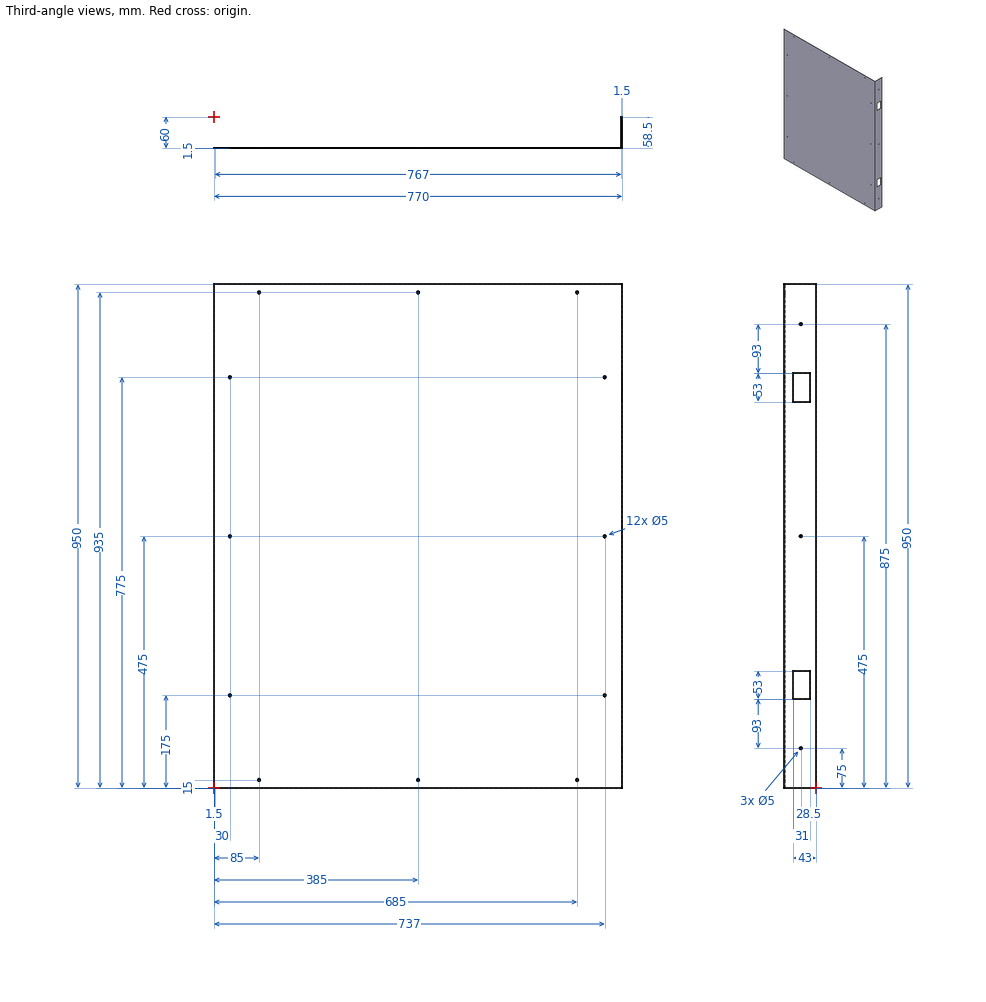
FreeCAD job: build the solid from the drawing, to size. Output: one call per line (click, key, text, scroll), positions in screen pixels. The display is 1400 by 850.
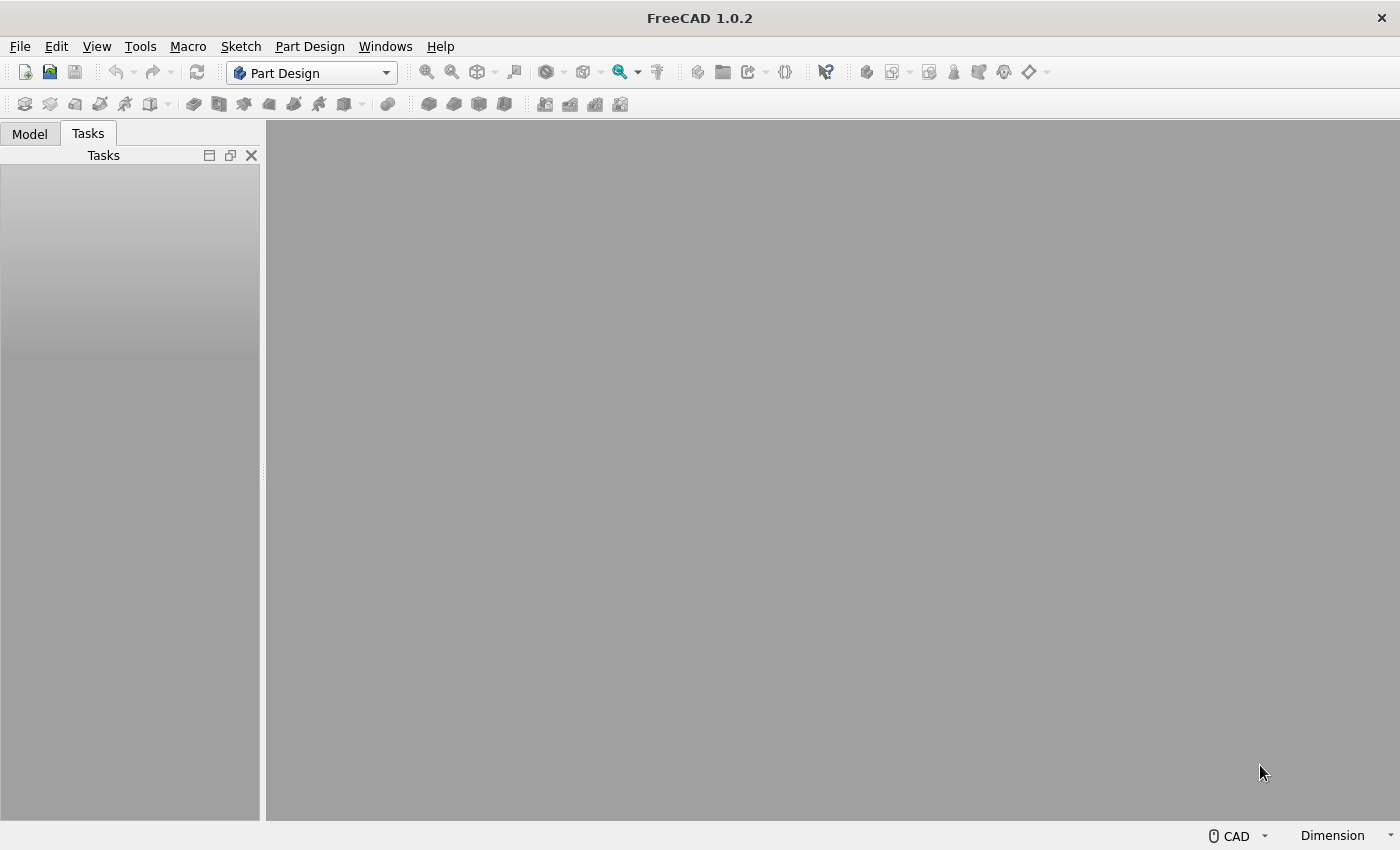
click(25, 72)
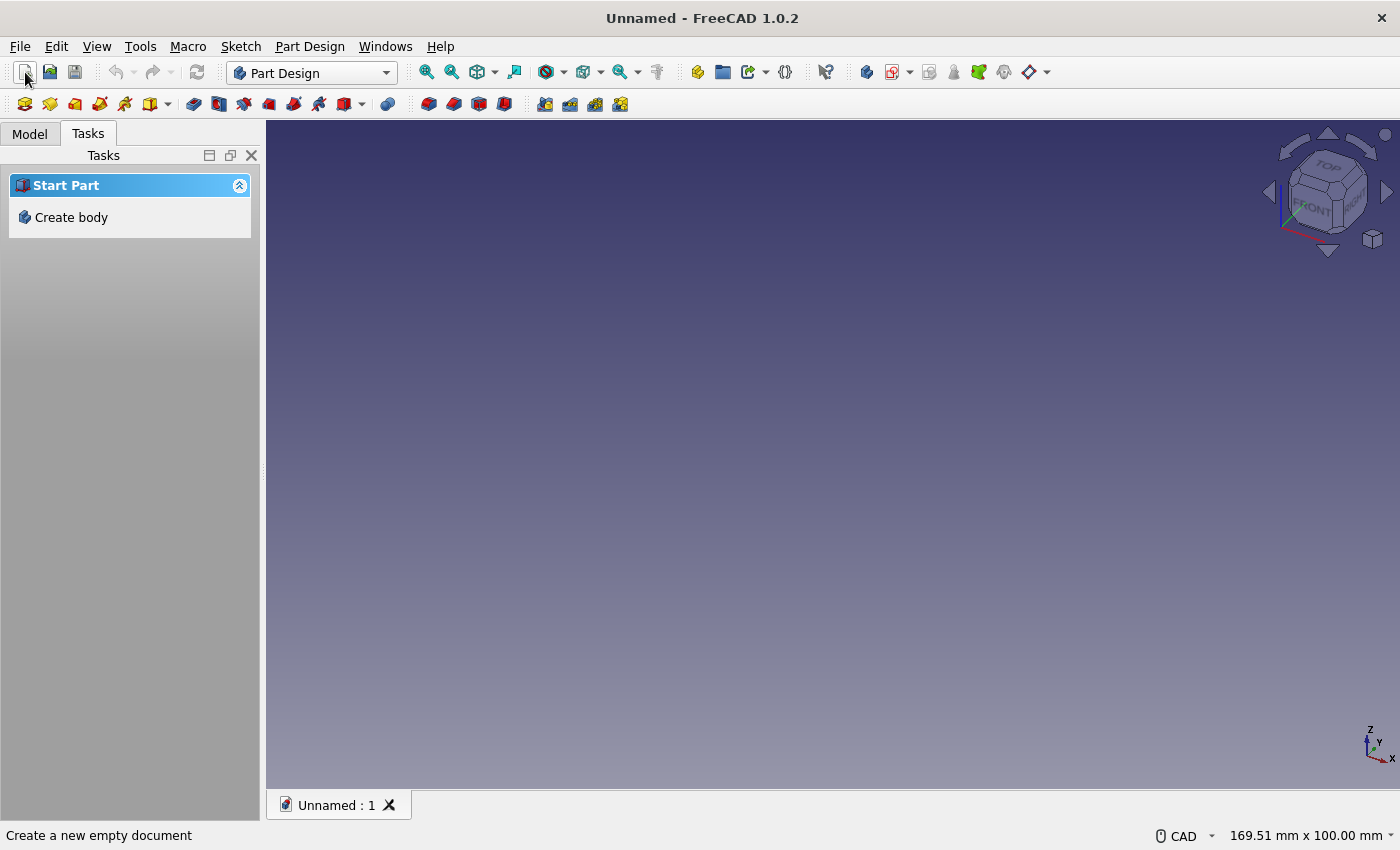
click(892, 72)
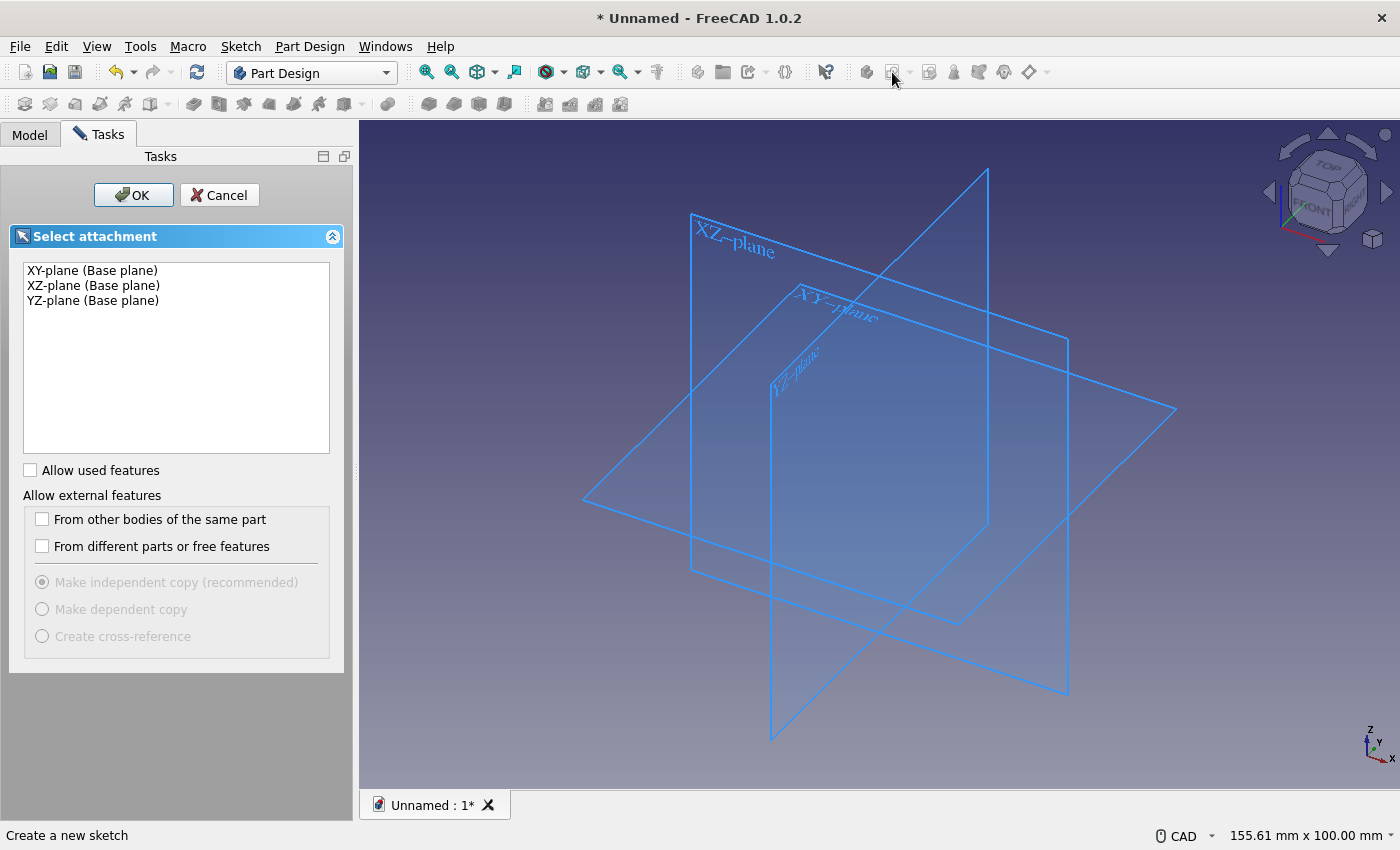
click(84, 270)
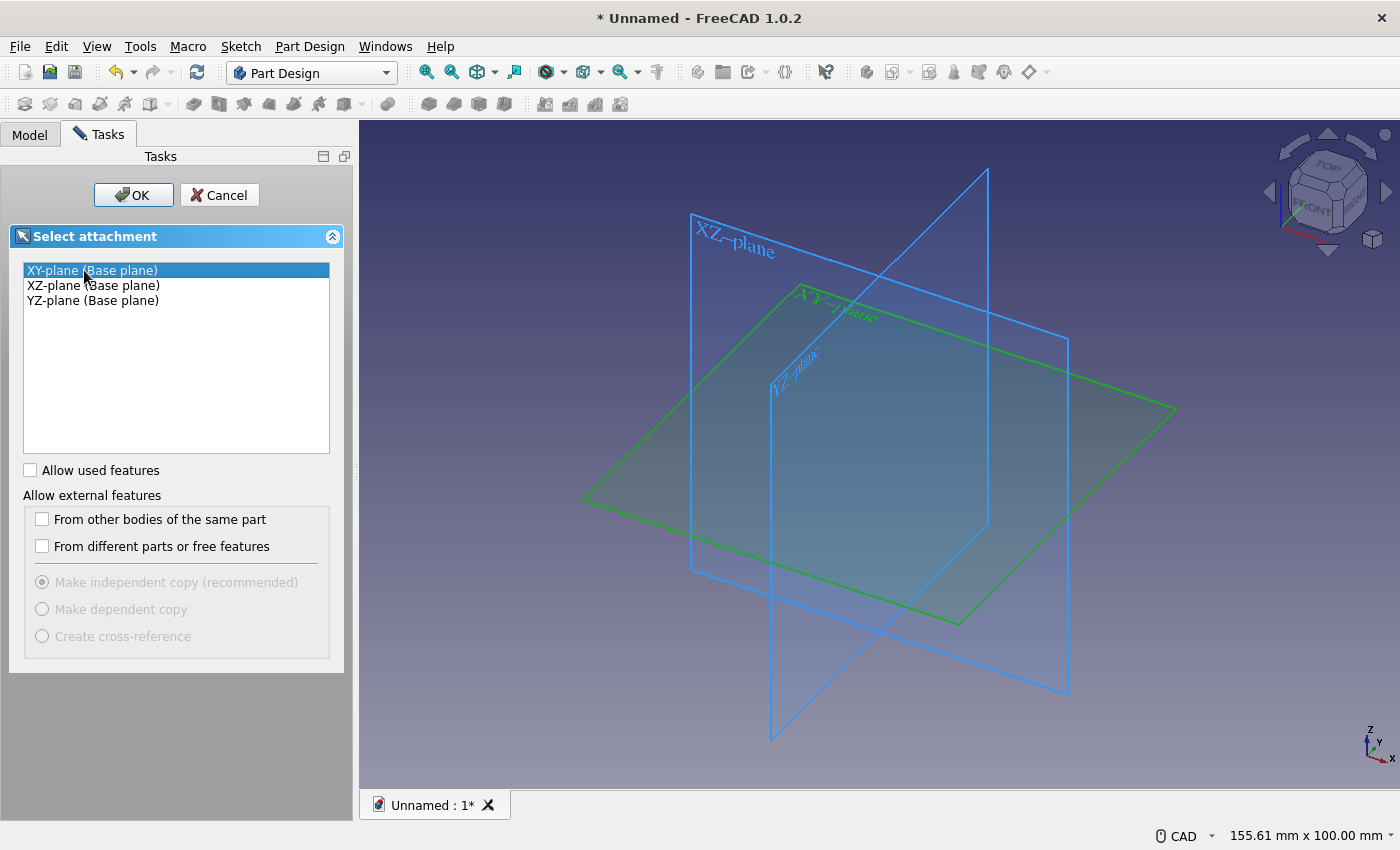
click(134, 195)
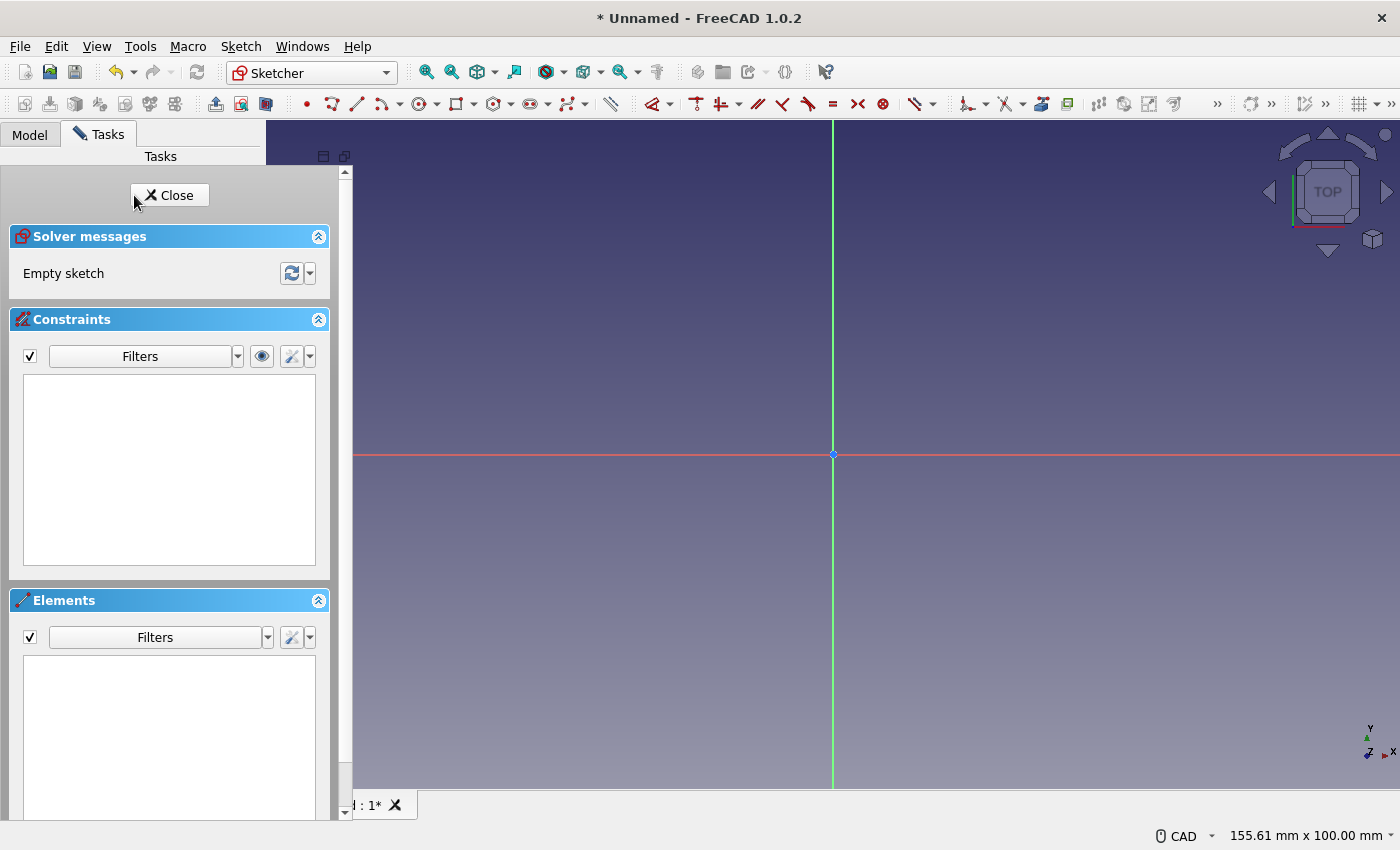
scroll(351, 423, down, 10)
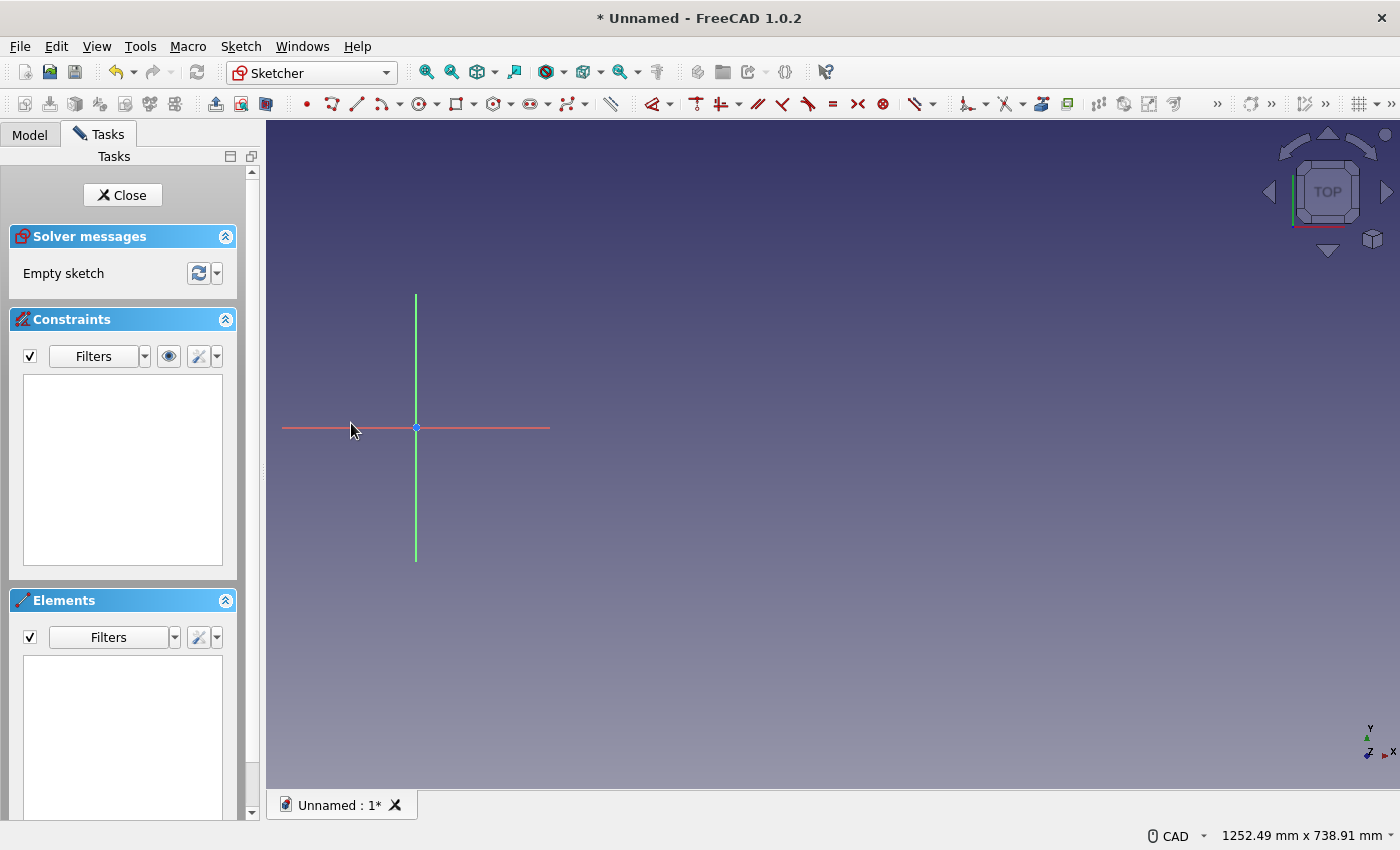
click(332, 104)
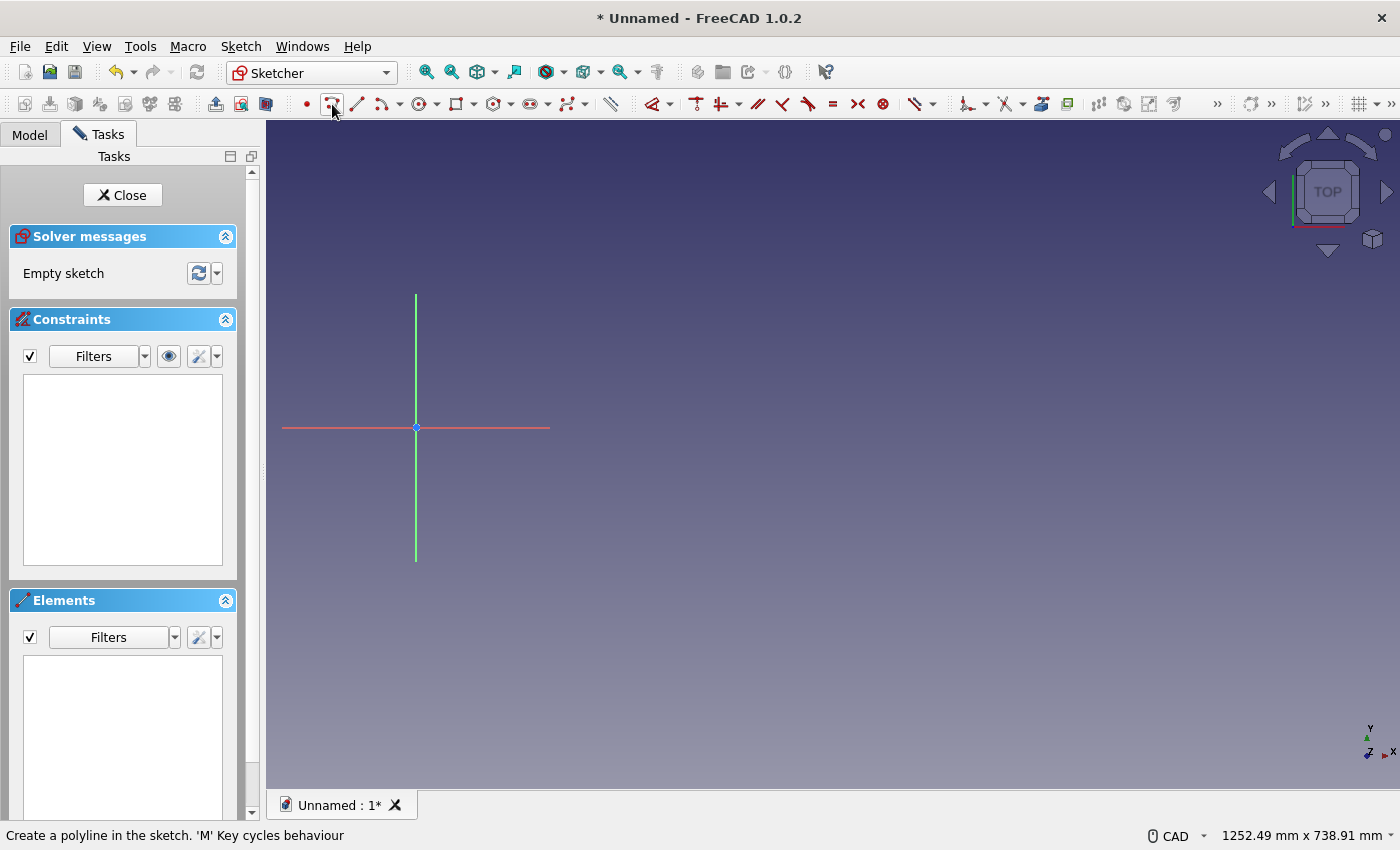
click(416, 428)
click(425, 482)
click(1113, 482)
click(1113, 428)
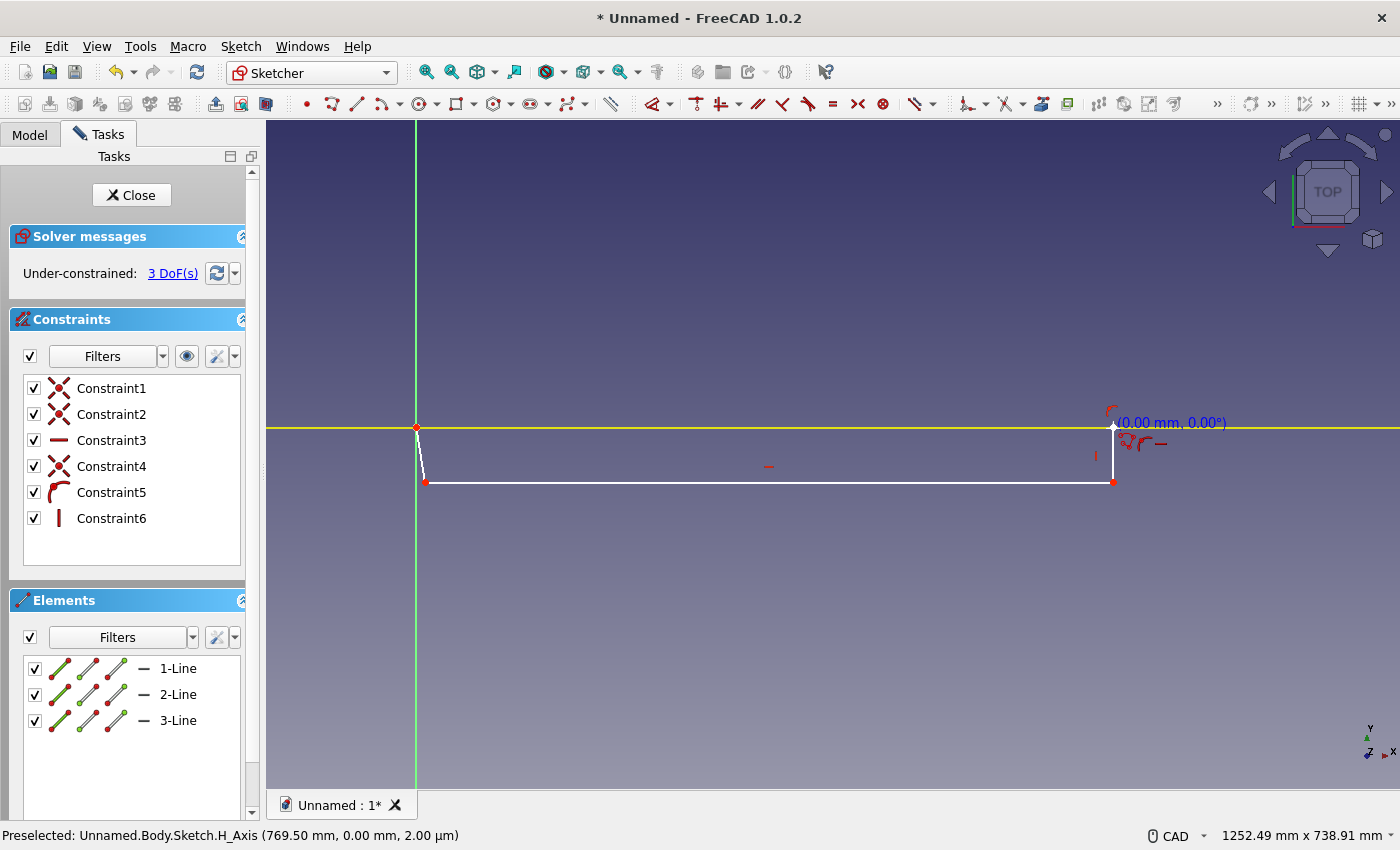
scroll(1112, 428, up, 13)